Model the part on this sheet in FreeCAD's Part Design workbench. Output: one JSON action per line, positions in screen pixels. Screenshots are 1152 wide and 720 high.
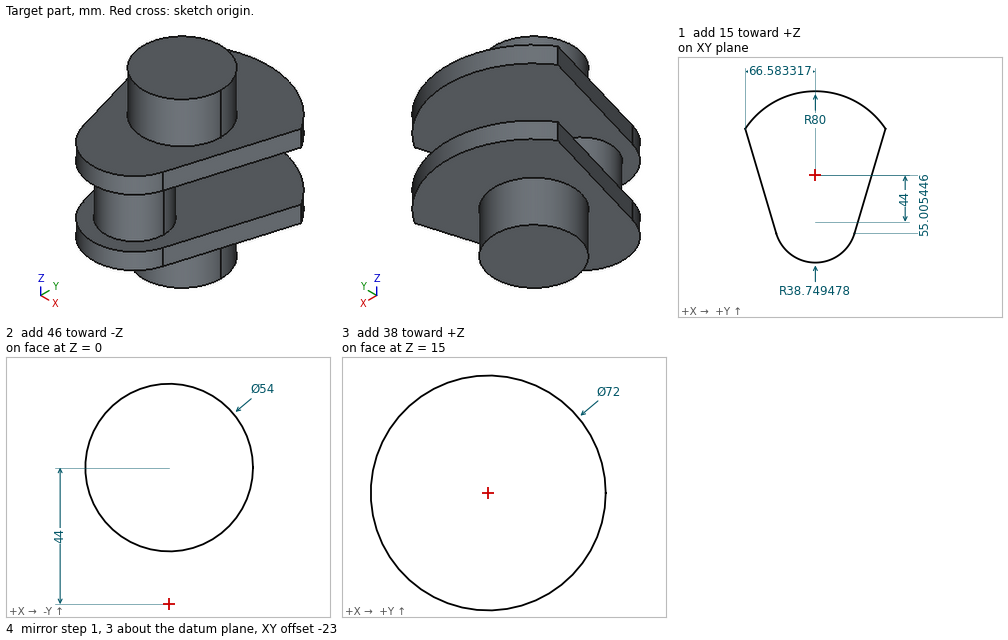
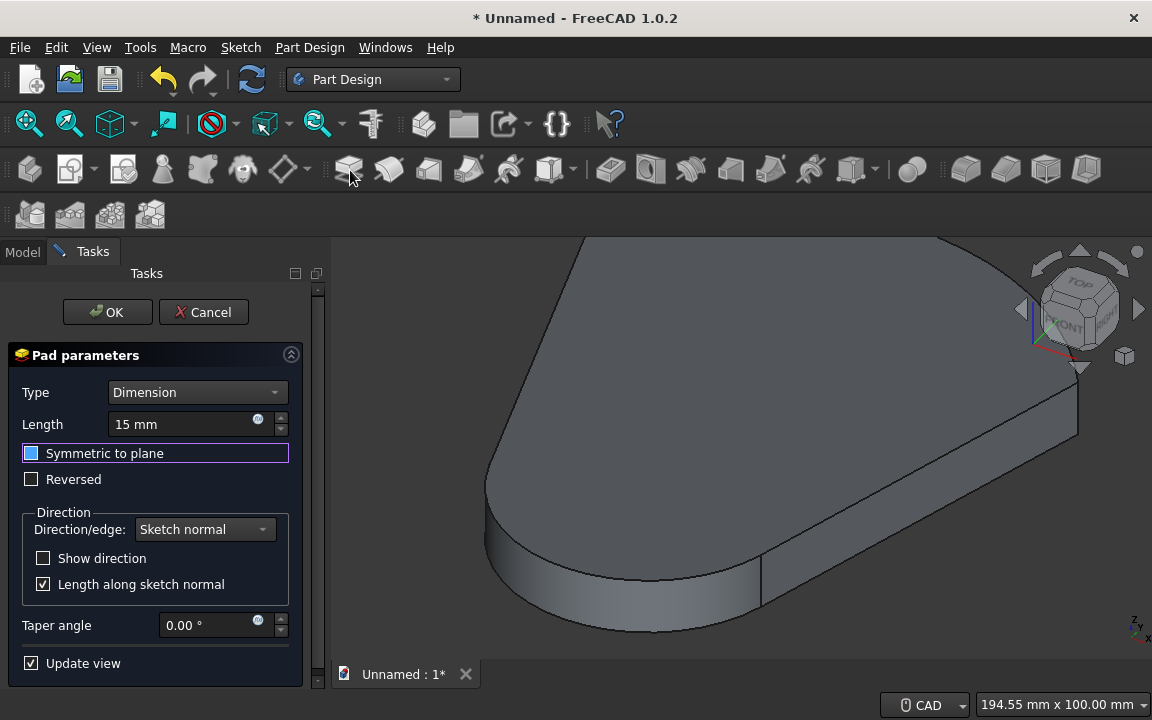
{"action": "left_click", "coordinate": [108, 312]}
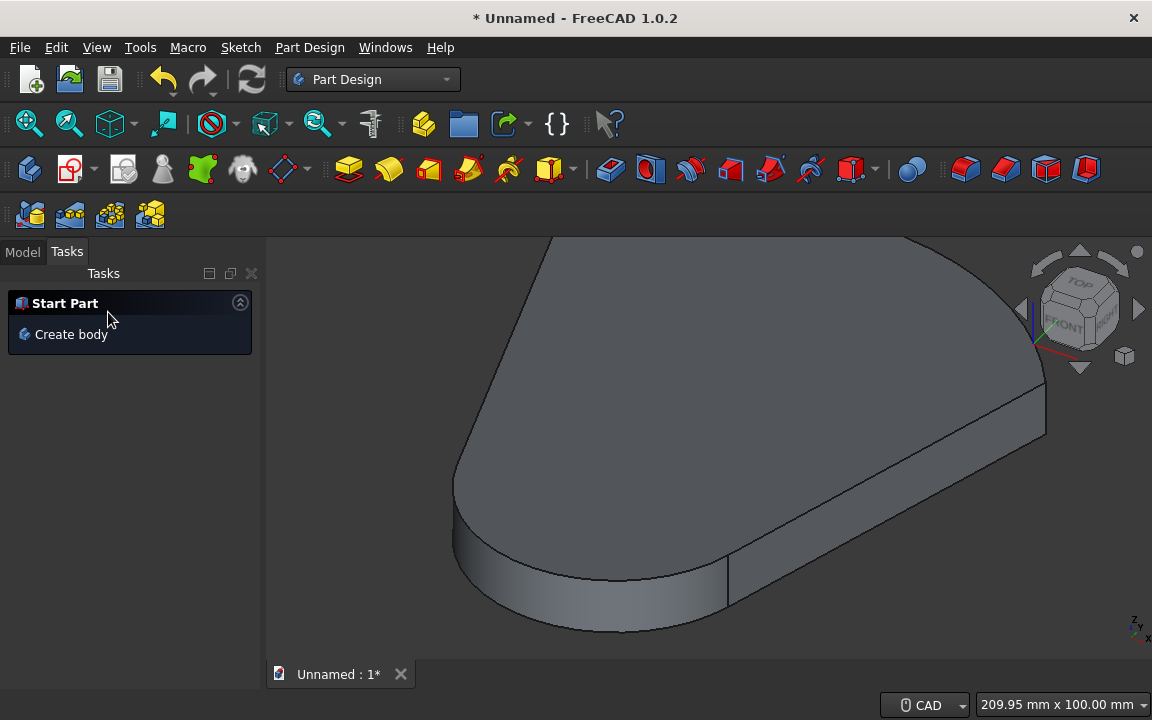
{"action": "left_click", "coordinate": [30, 124]}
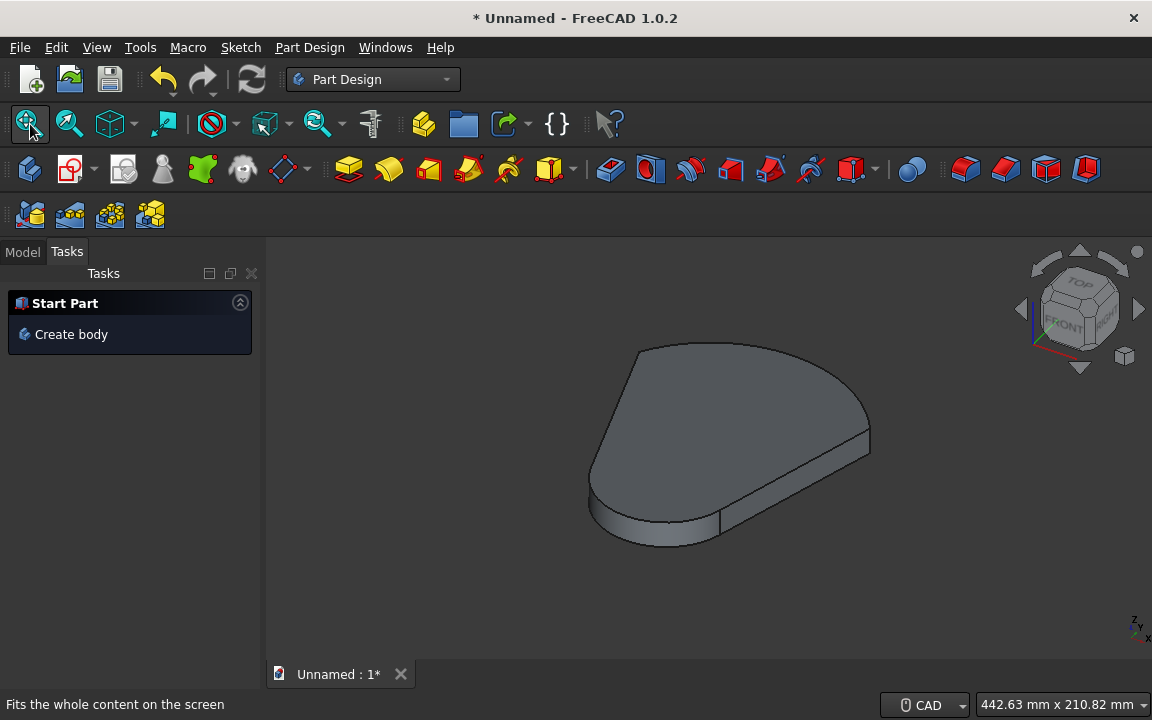
{"action": "key", "text": "5"}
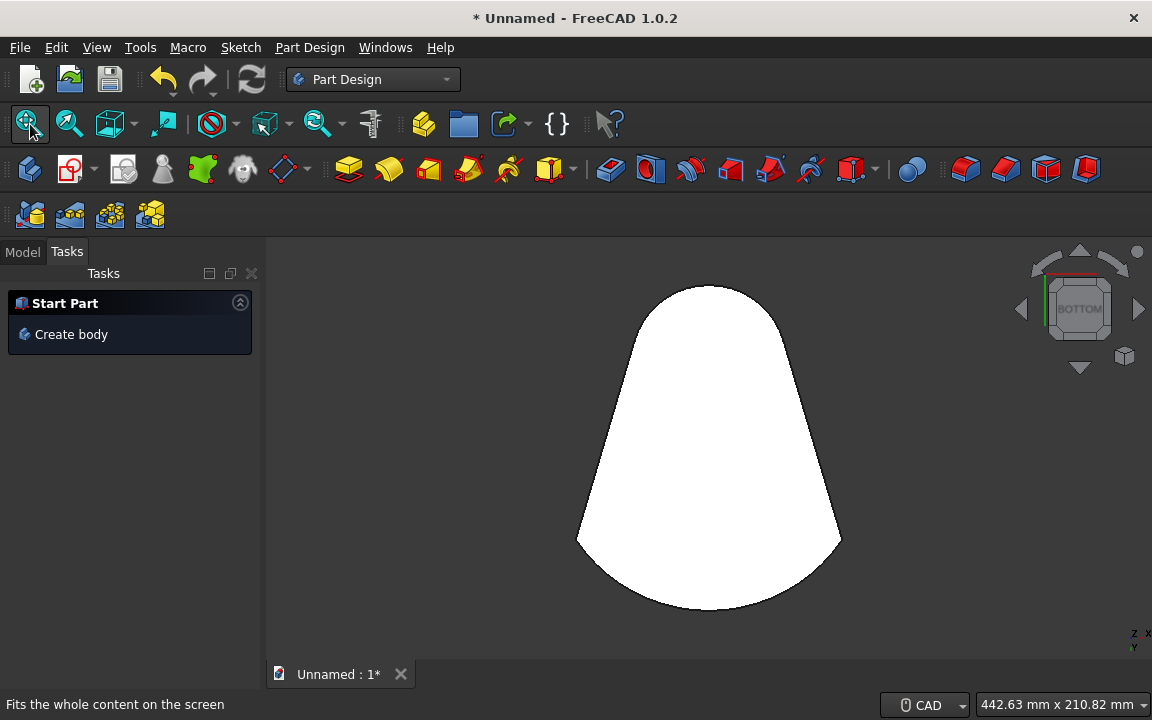
{"action": "left_click", "coordinate": [709, 494]}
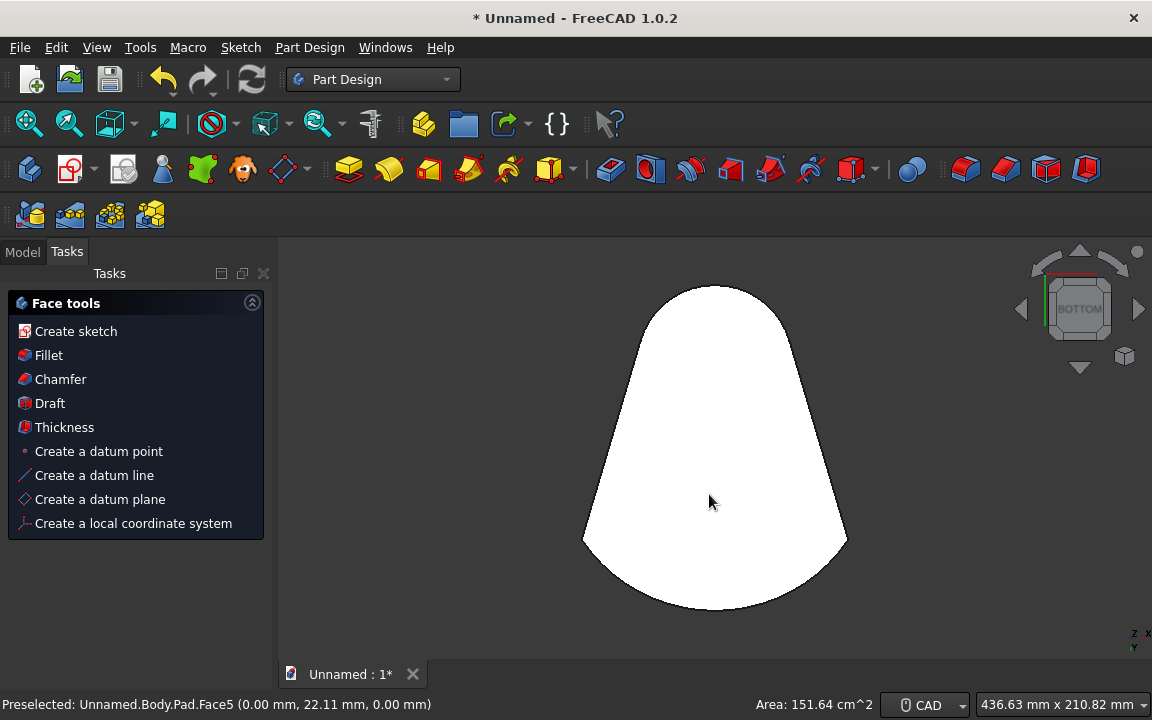
{"action": "left_click", "coordinate": [70, 170]}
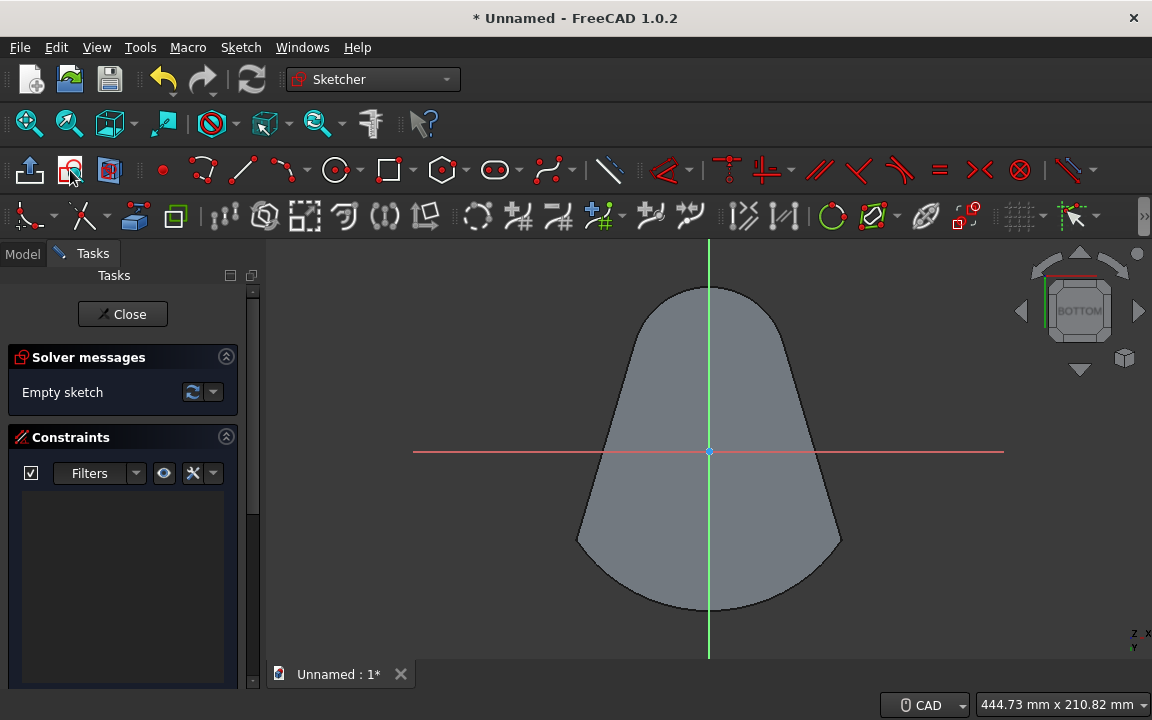
{"action": "scroll", "coordinate": [792, 298], "scroll_direction": "up", "scroll_amount": 3}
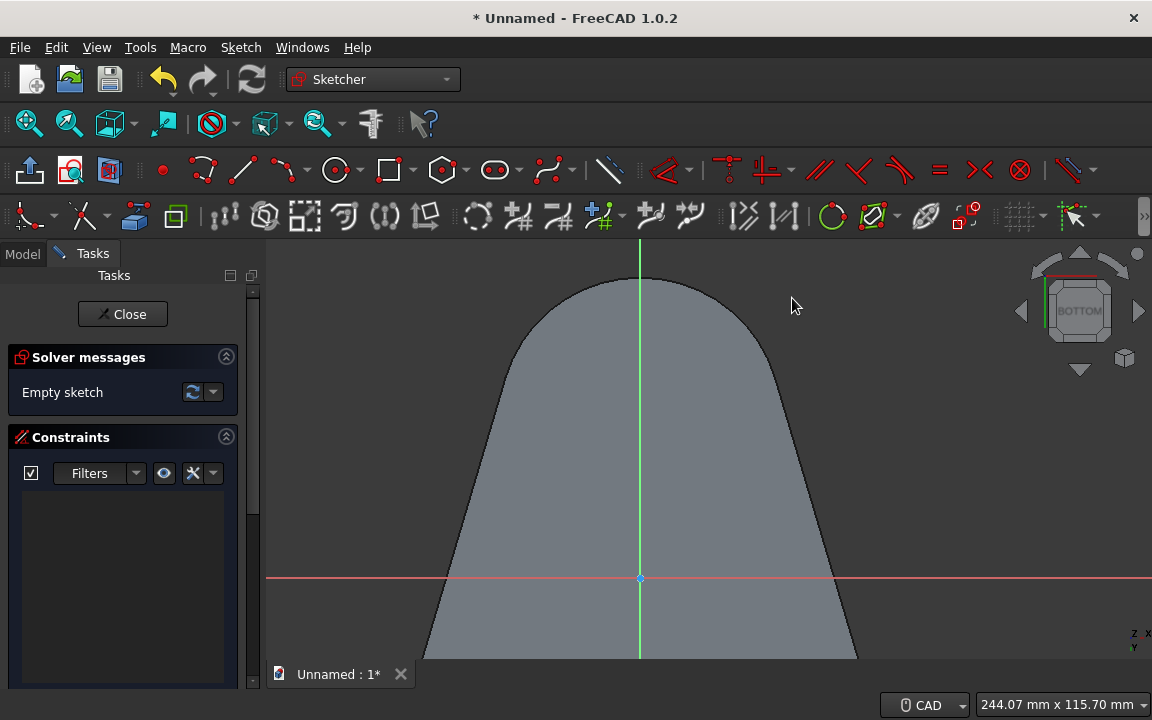
{"action": "left_click", "coordinate": [336, 170]}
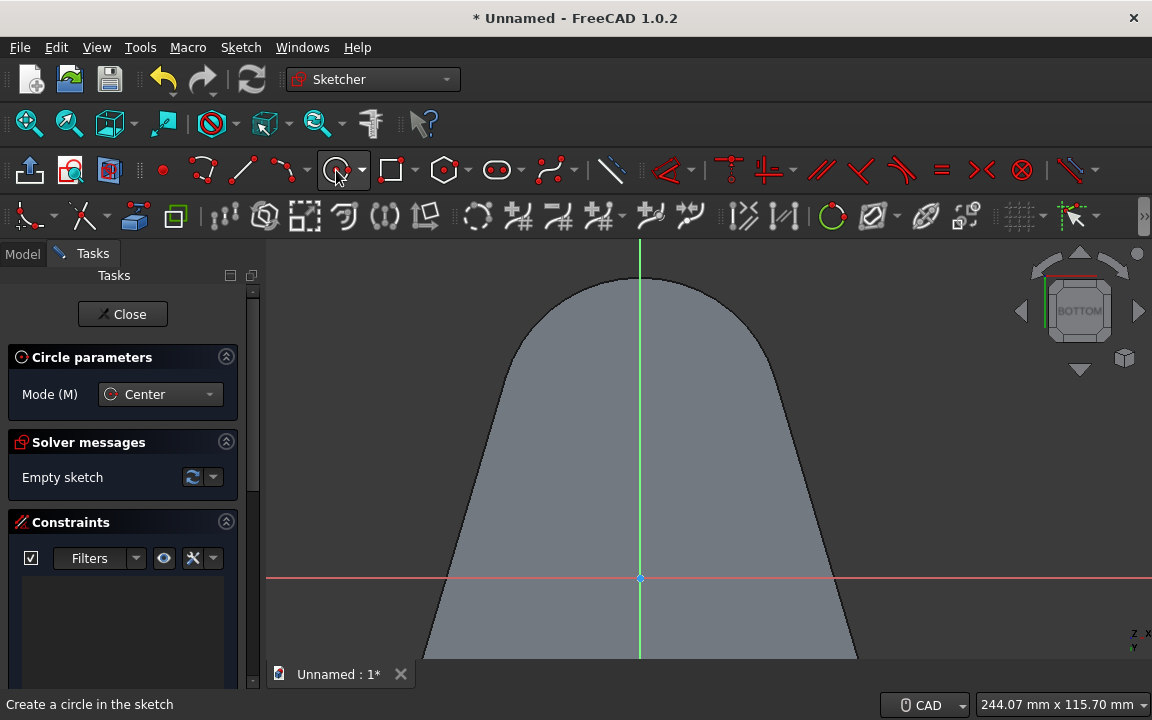
{"action": "left_click", "coordinate": [640, 418]}
{"action": "left_click", "coordinate": [710, 349]}
{"action": "key", "text": "Escape"}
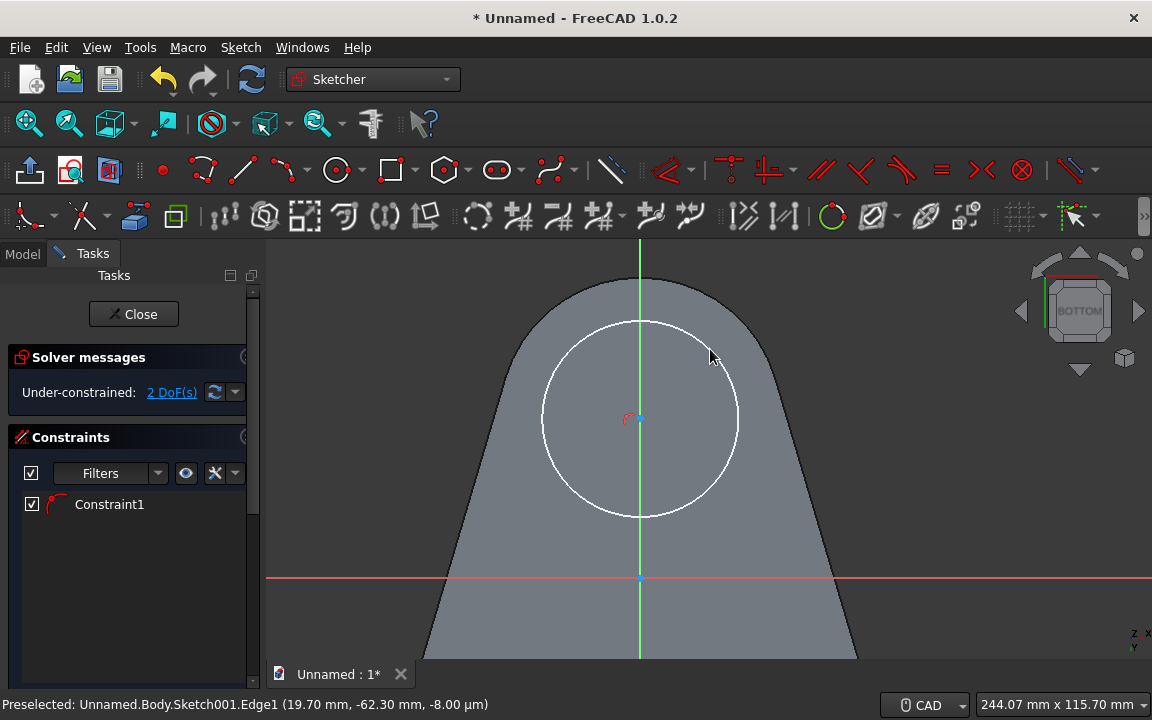
{"action": "left_click", "coordinate": [666, 170]}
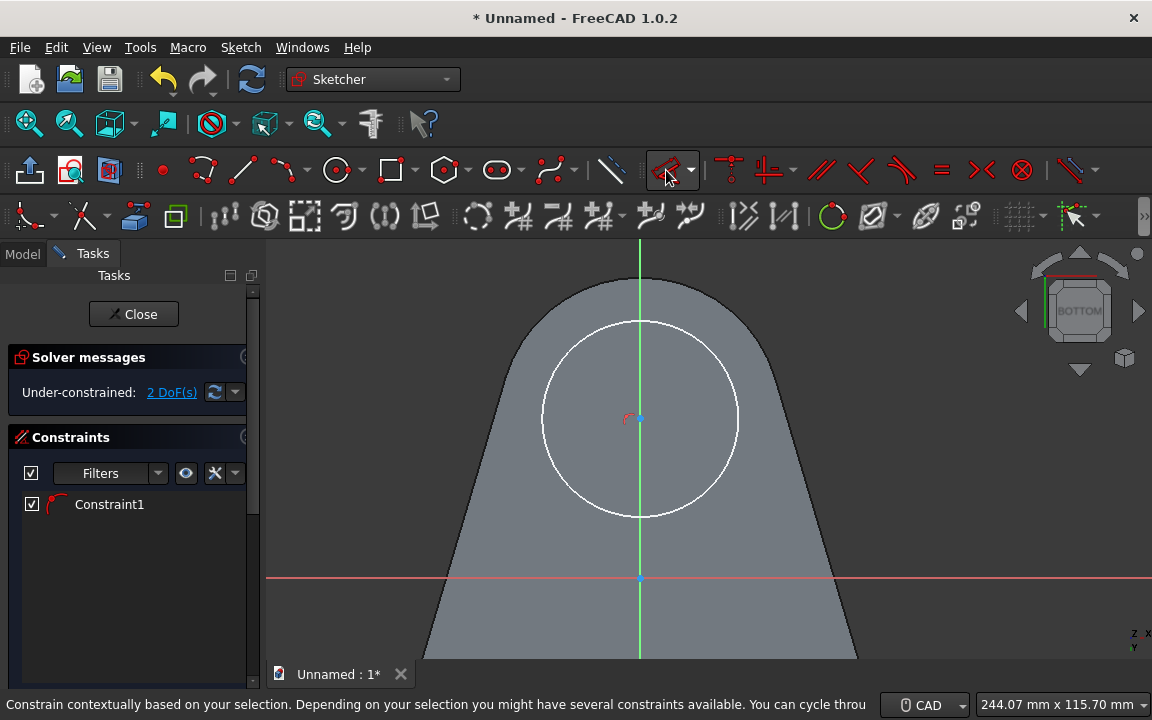
{"action": "left_click", "coordinate": [709, 349]}
{"action": "left_click", "coordinate": [731, 326]}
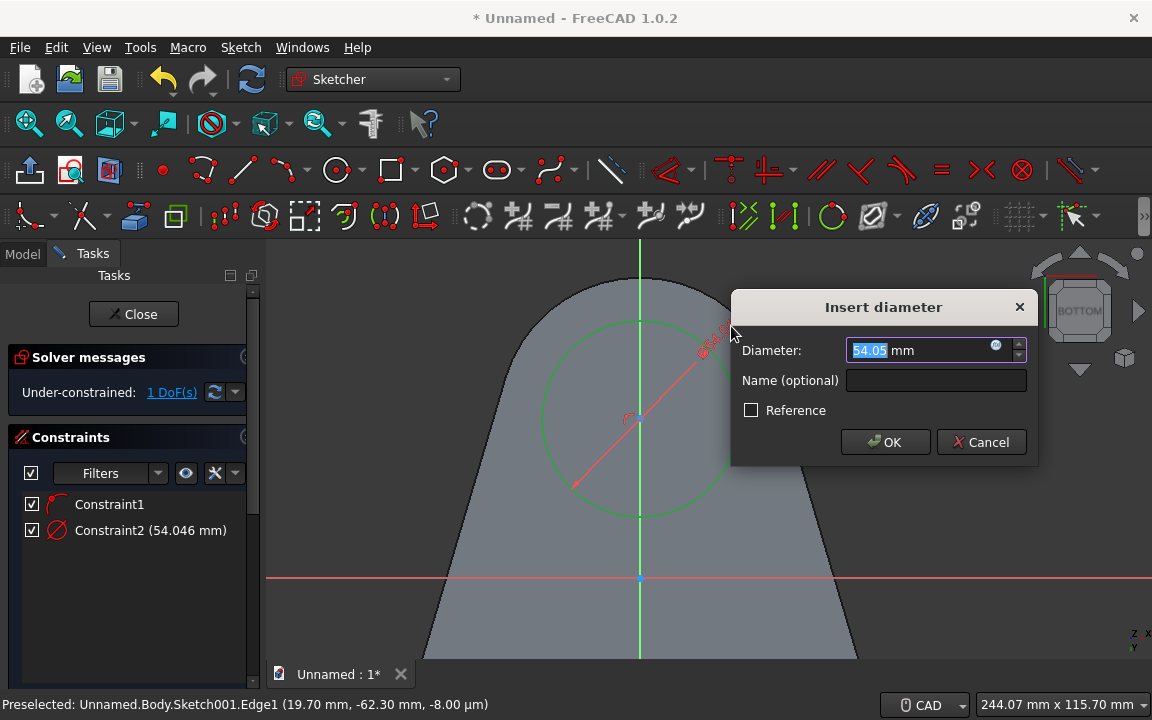
{"action": "type", "text": "54"}
{"action": "key", "text": "Return"}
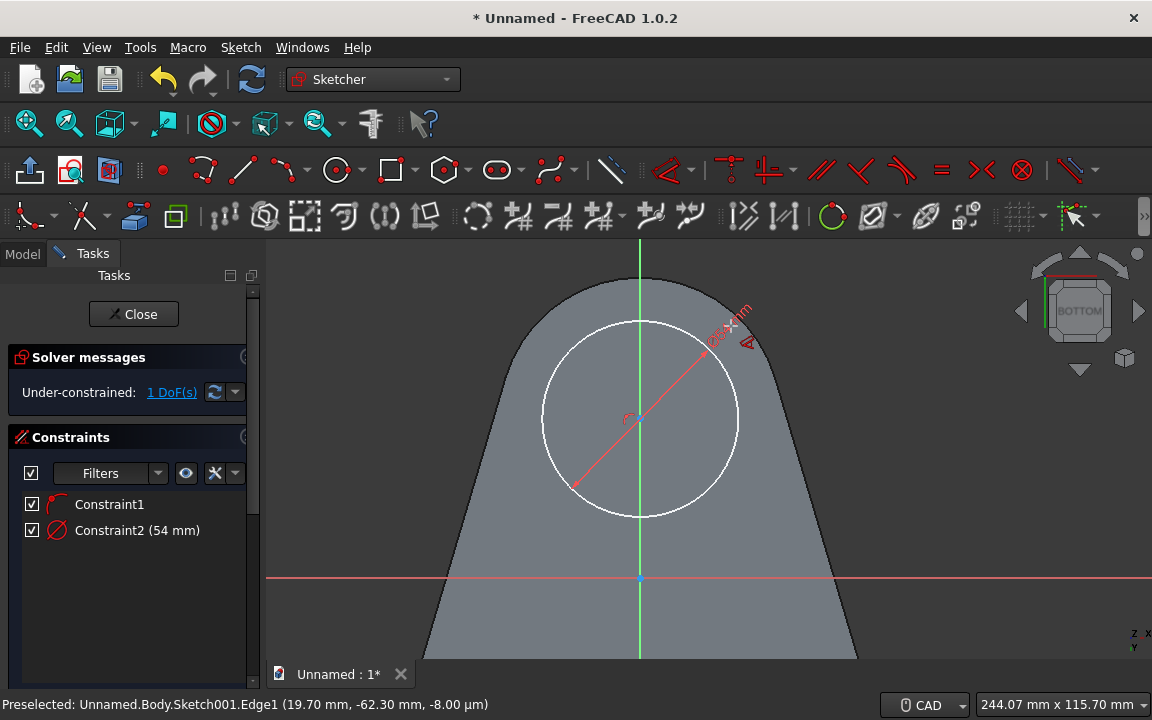
{"action": "left_click", "coordinate": [640, 419]}
{"action": "left_click", "coordinate": [674, 462]}